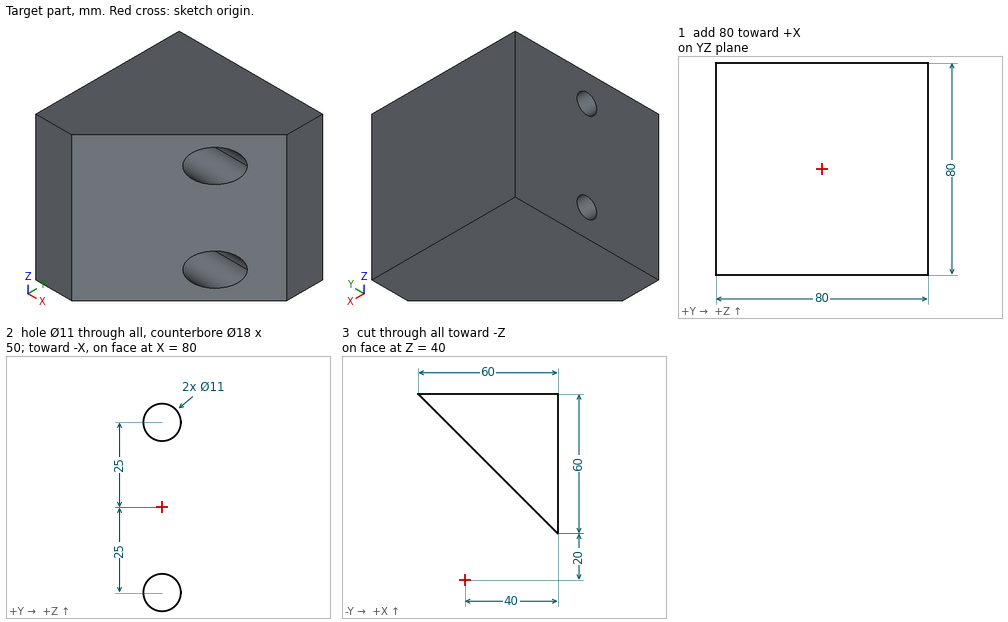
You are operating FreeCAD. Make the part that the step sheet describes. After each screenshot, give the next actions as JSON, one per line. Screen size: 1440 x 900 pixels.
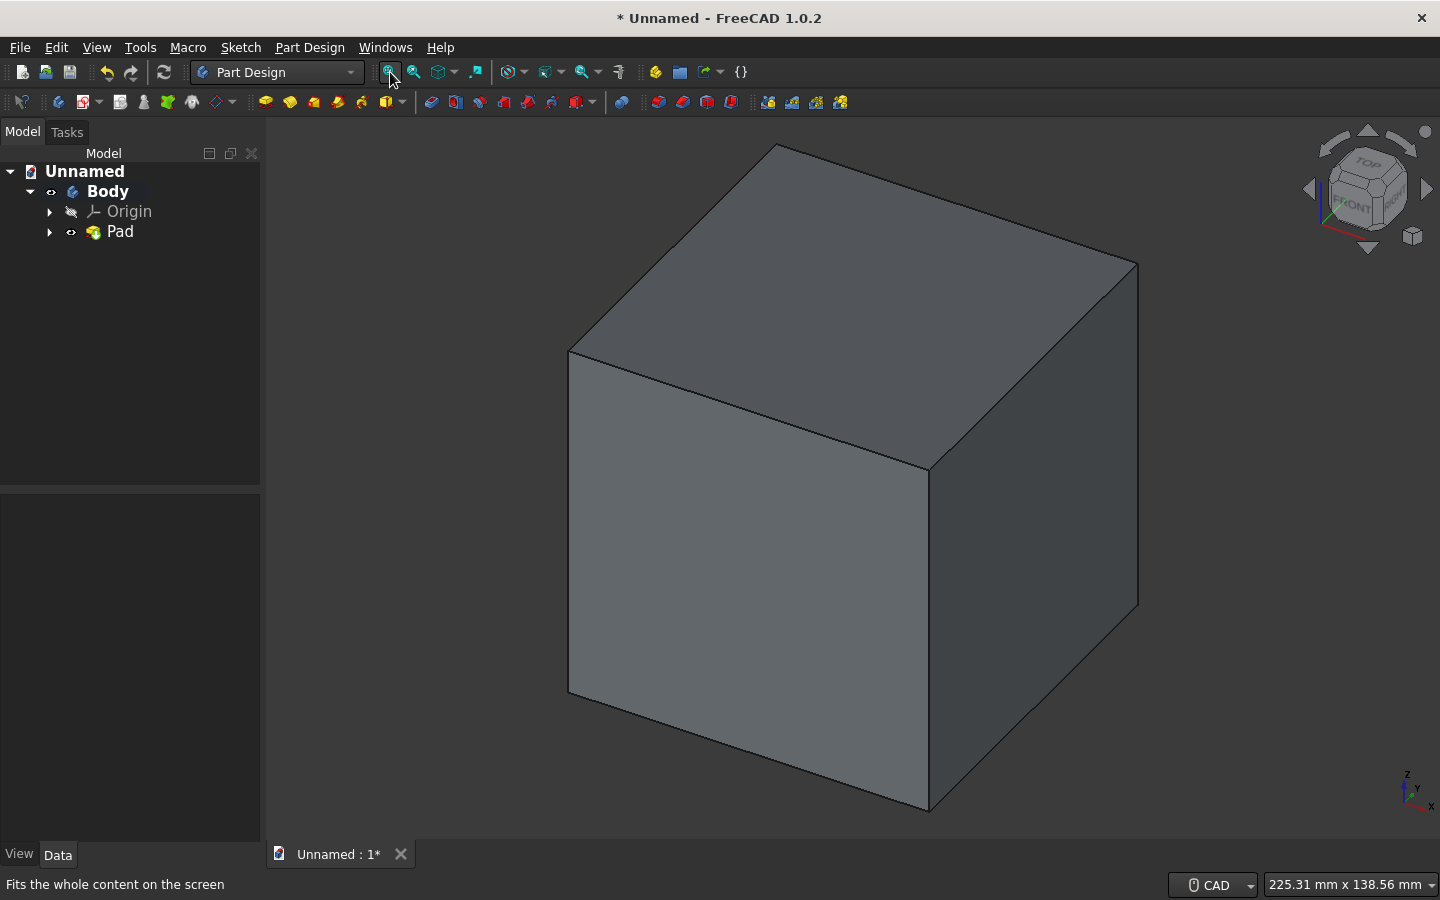
{"action": "left_click", "coordinate": [1034, 537]}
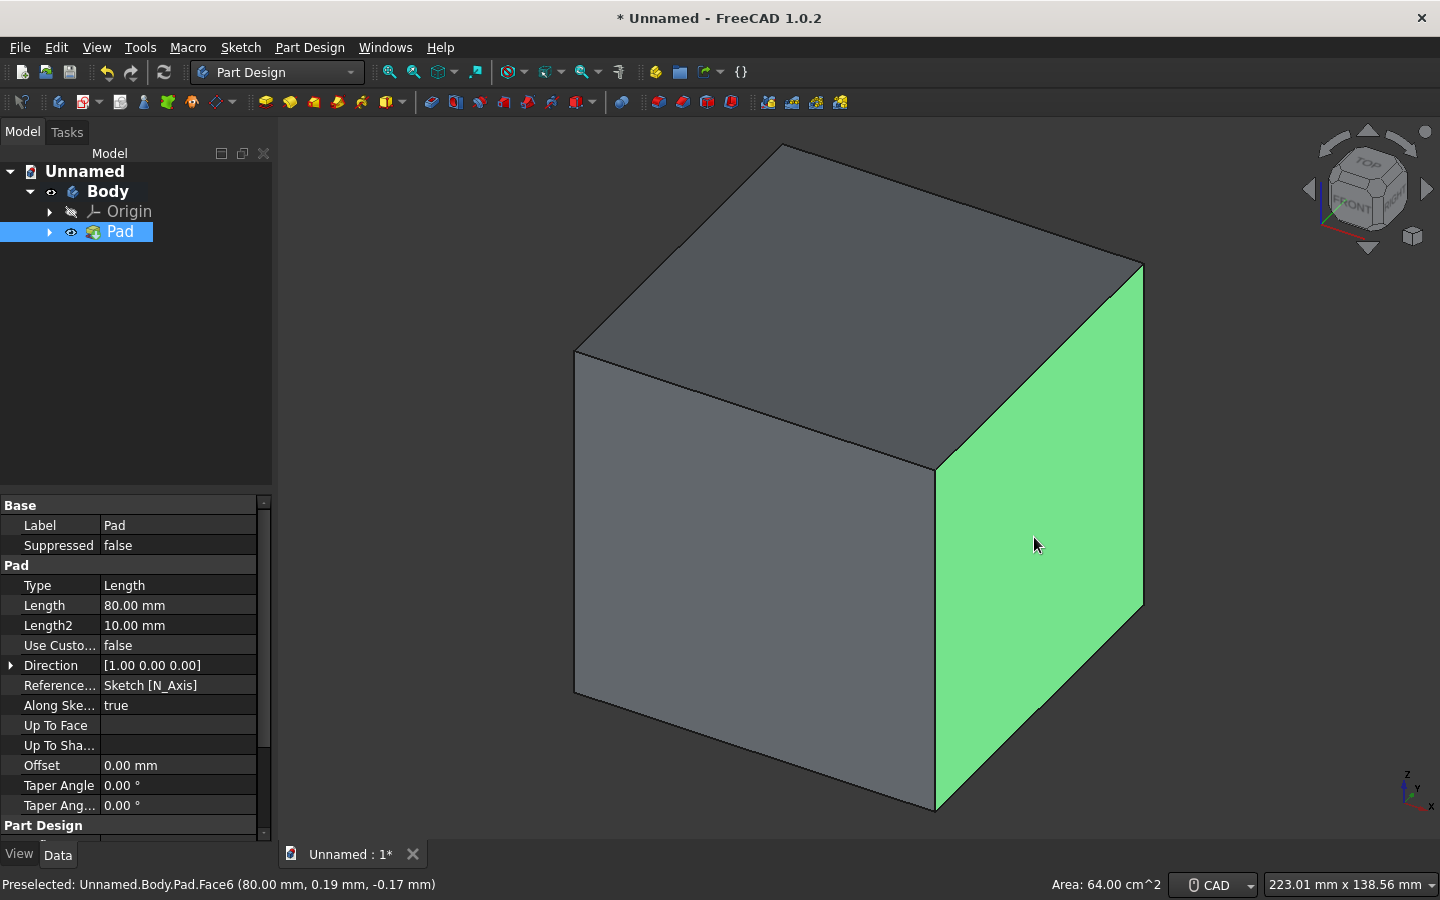
{"action": "left_click", "coordinate": [84, 102]}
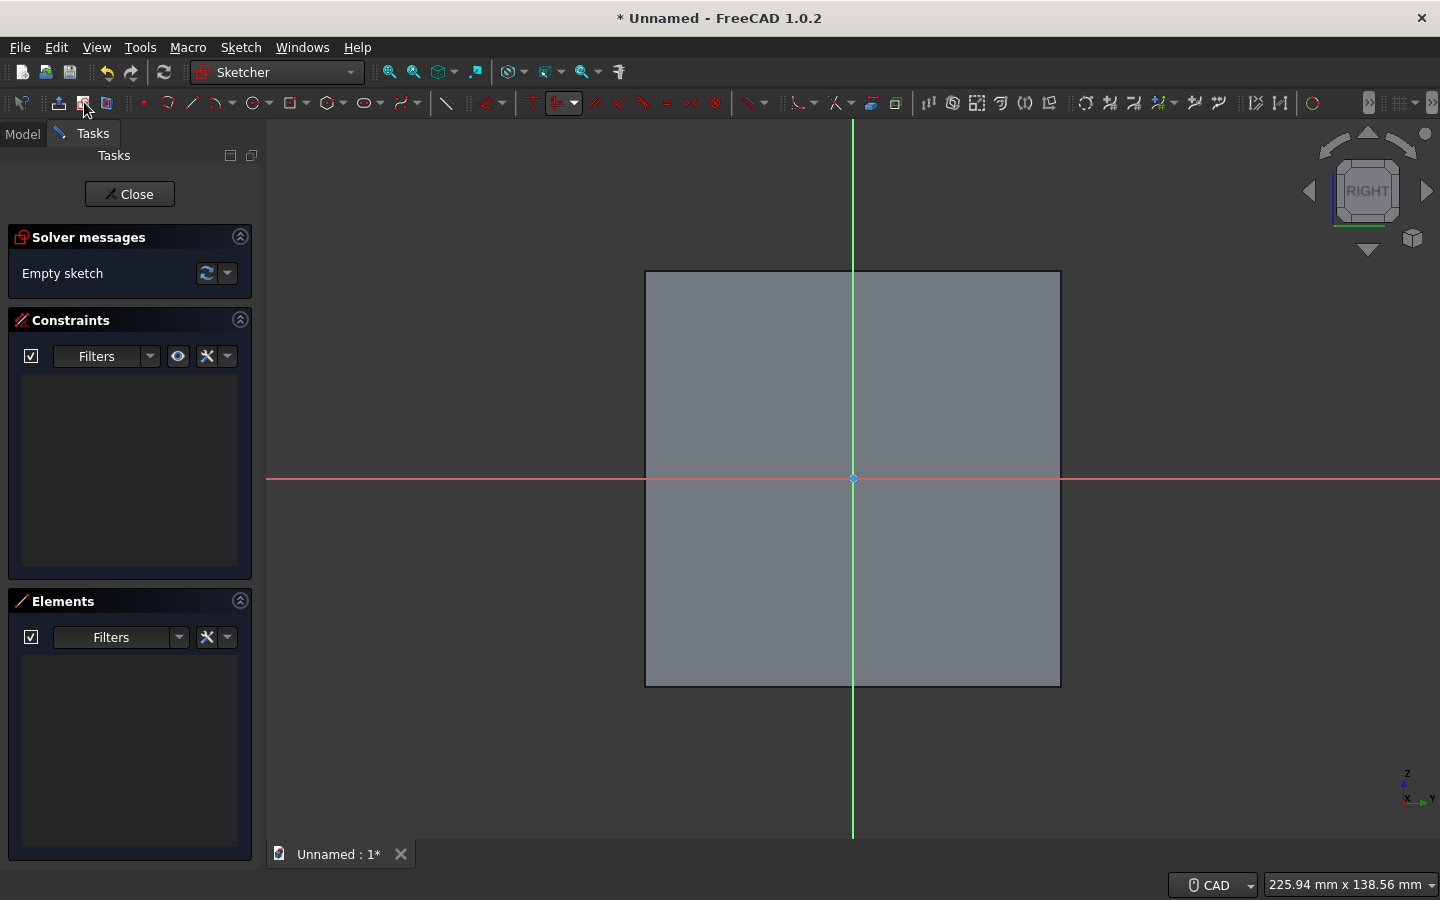
{"action": "scroll", "coordinate": [992, 479], "scroll_direction": "up", "scroll_amount": 2}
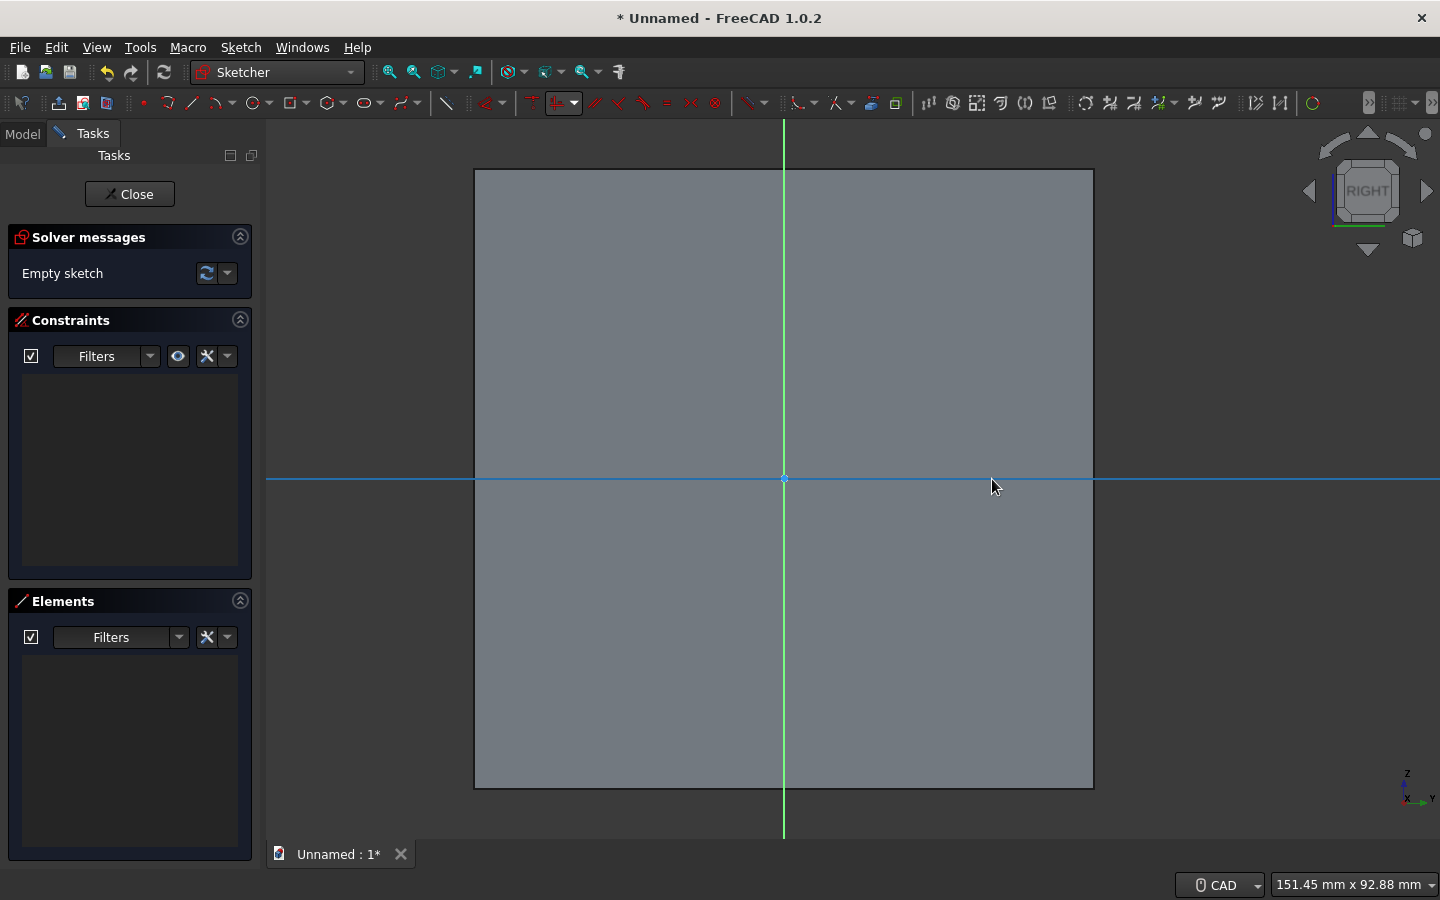
{"action": "left_click", "coordinate": [254, 104]}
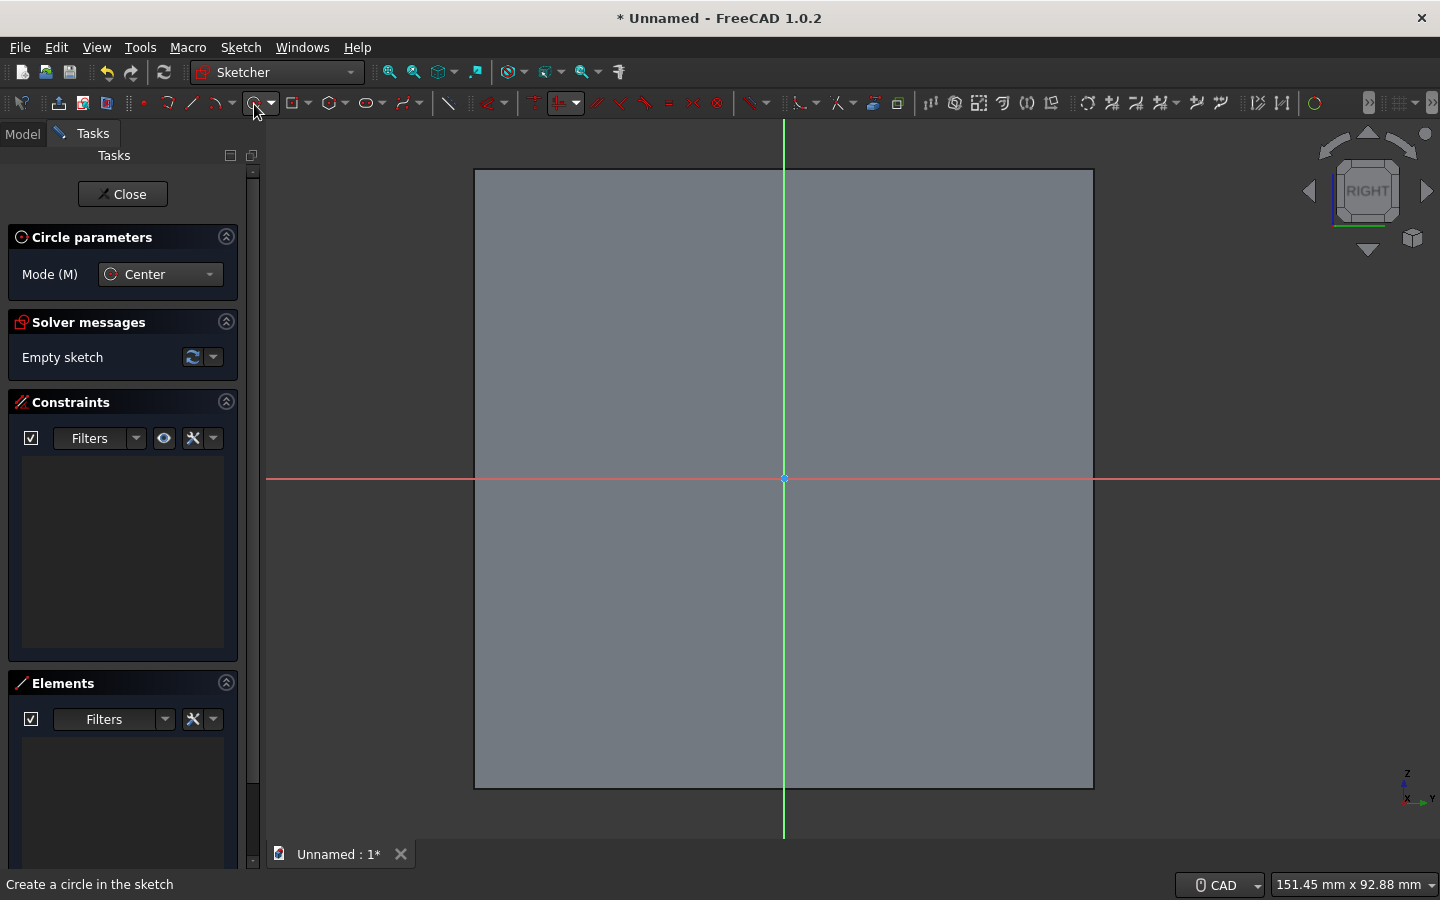
{"action": "left_click", "coordinate": [784, 285]}
{"action": "left_click", "coordinate": [814, 255]}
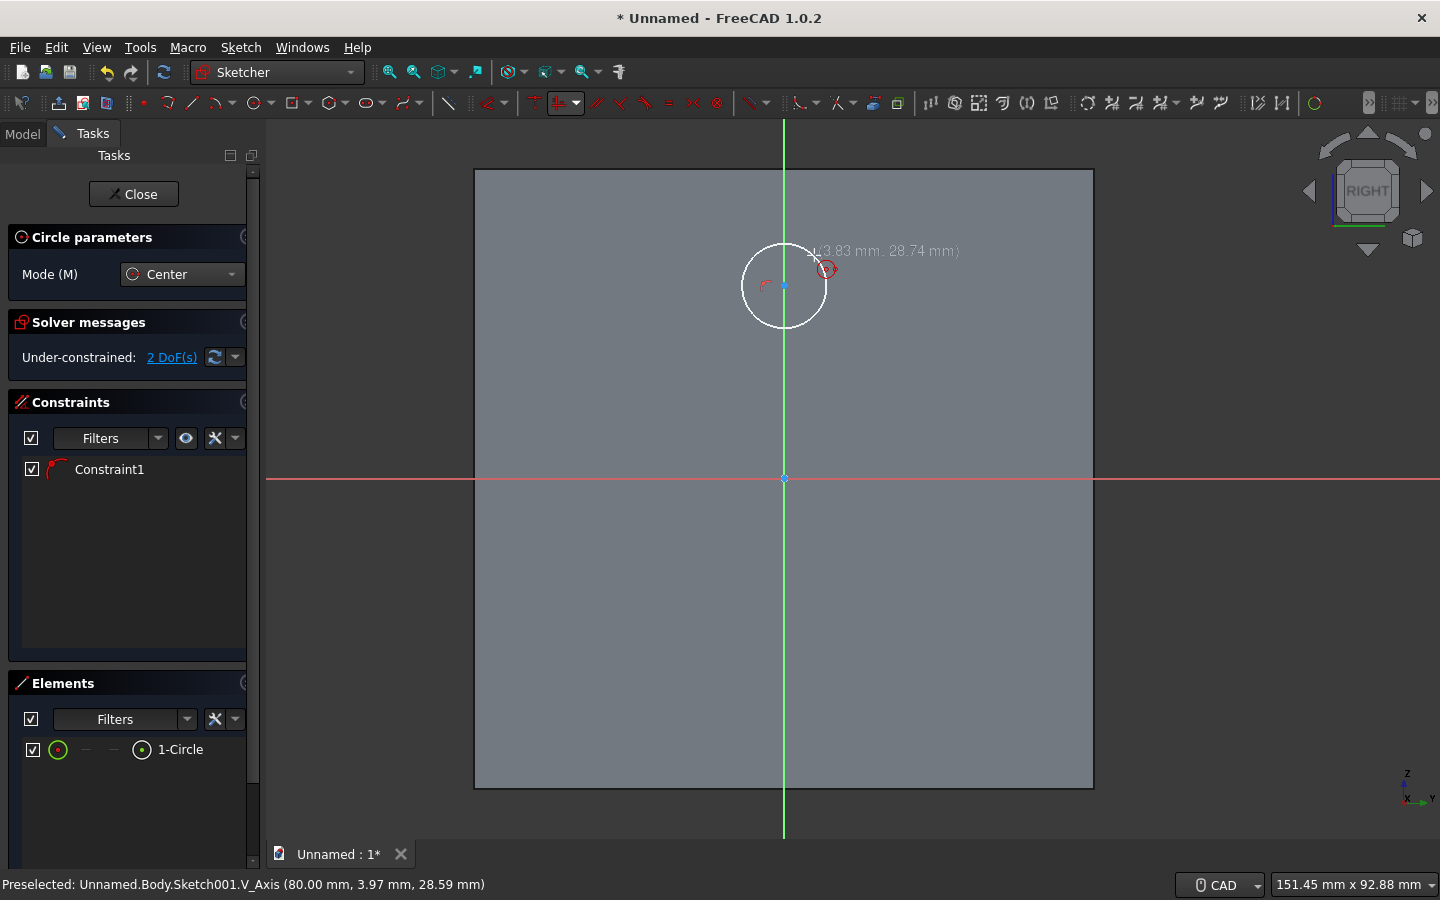
{"action": "left_click", "coordinate": [784, 673]}
{"action": "left_click", "coordinate": [814, 642]}
{"action": "key", "text": "Escape"}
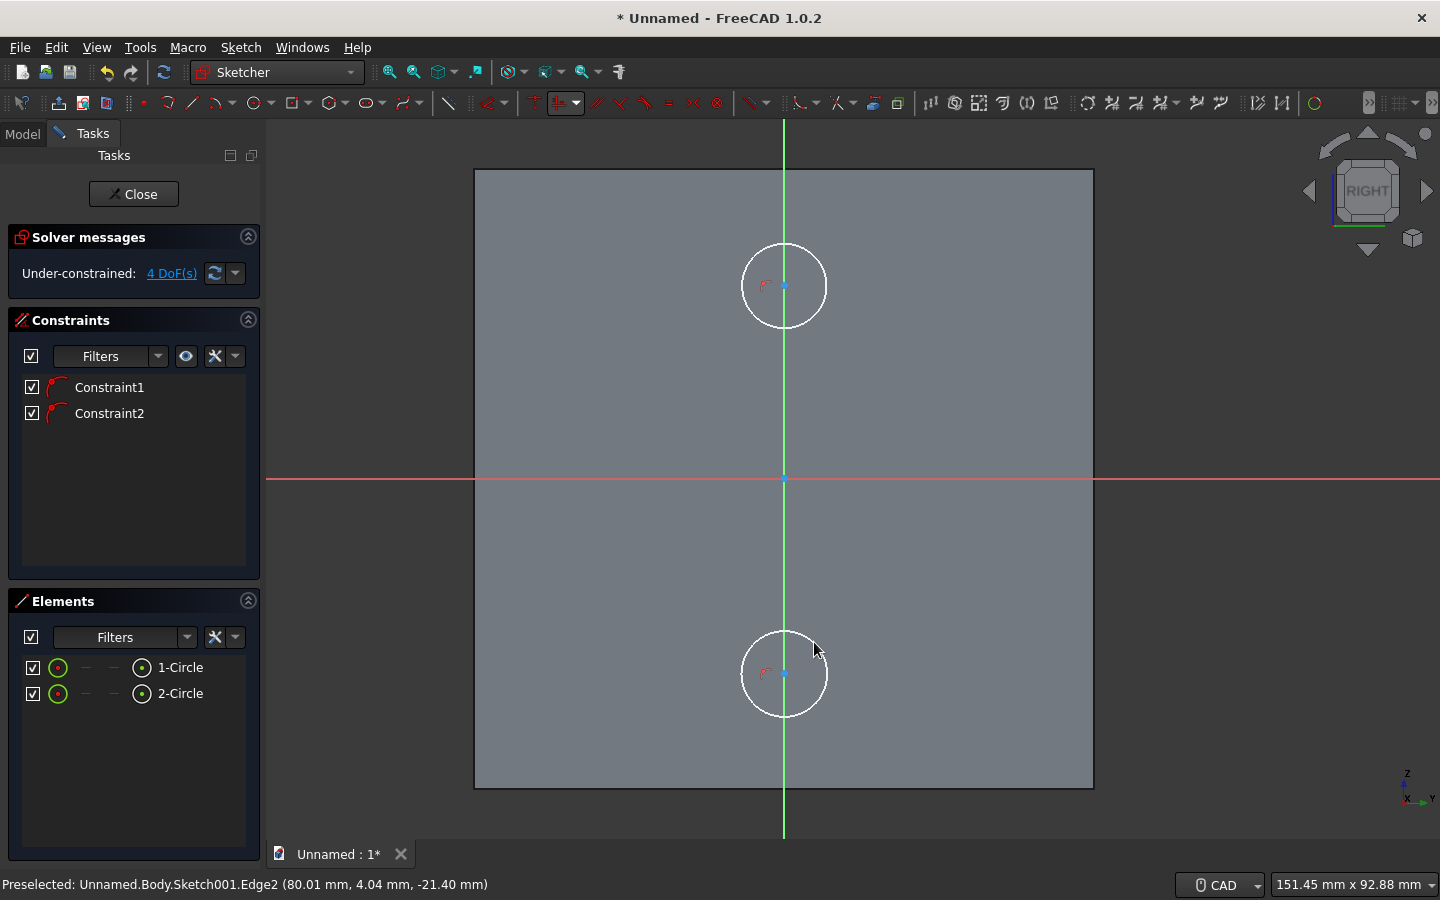
{"action": "left_click", "coordinate": [814, 256]}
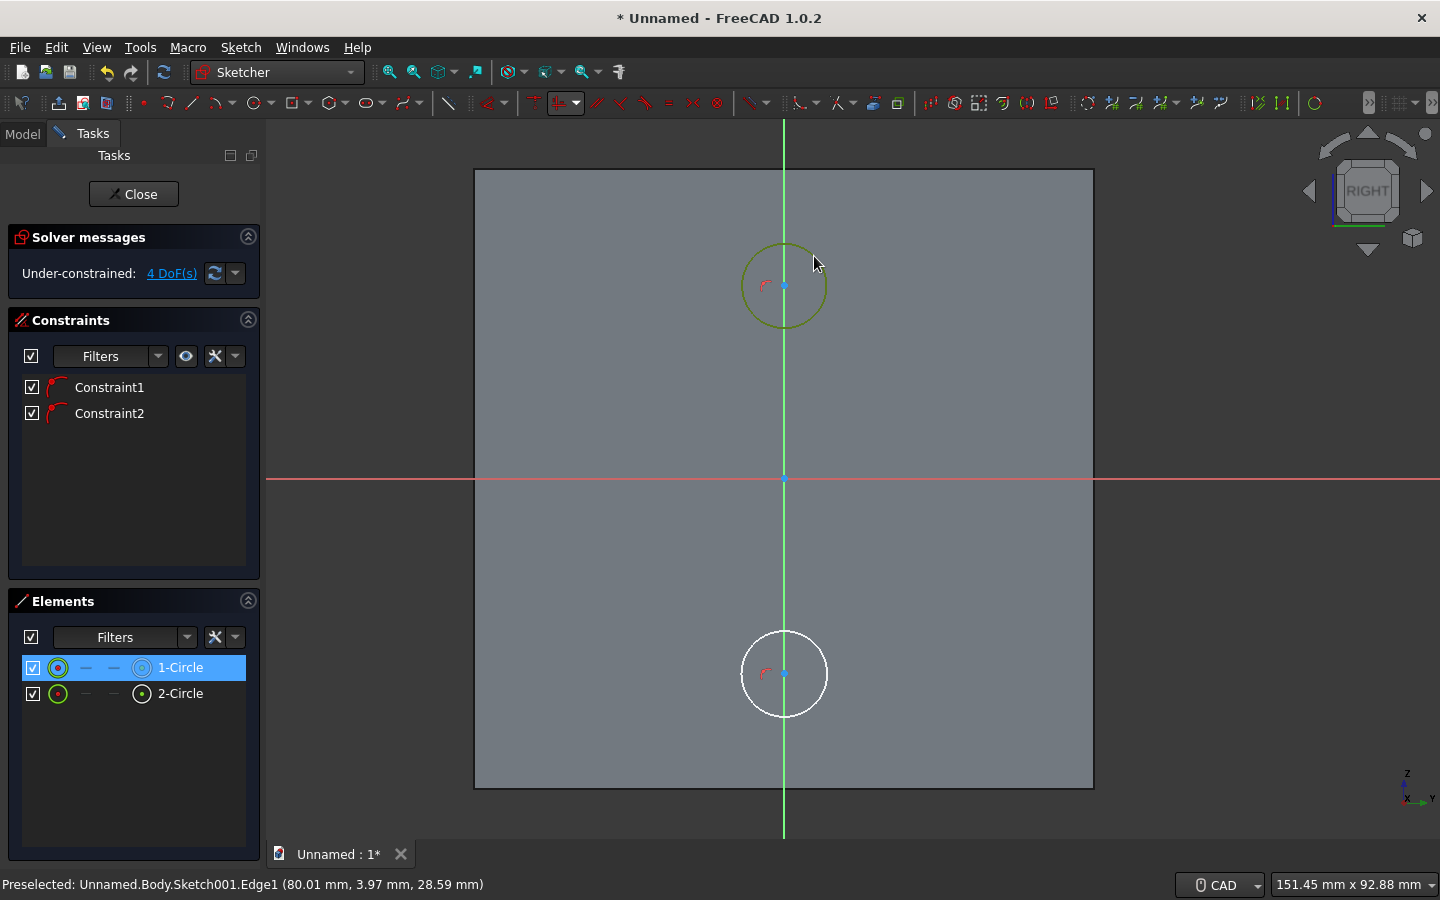
{"action": "left_click", "coordinate": [815, 644]}